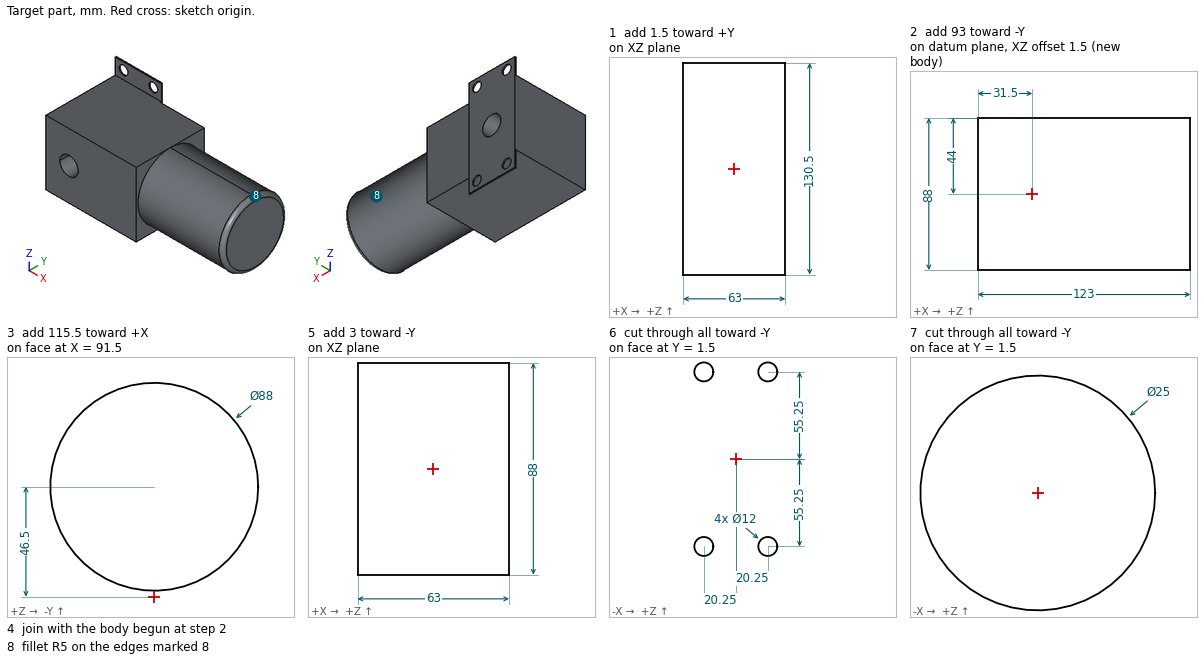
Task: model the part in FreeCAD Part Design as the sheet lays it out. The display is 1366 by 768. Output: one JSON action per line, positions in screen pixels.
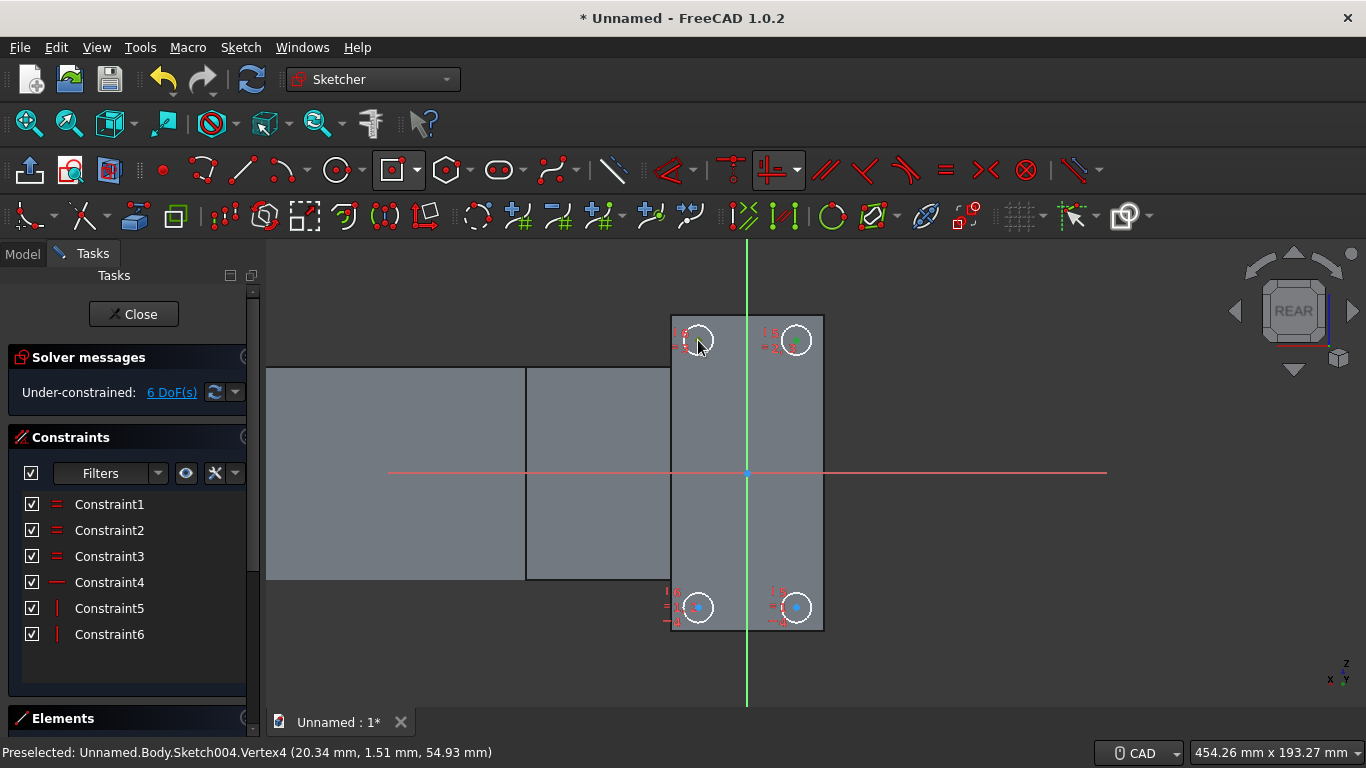
{"action": "key", "text": "h"}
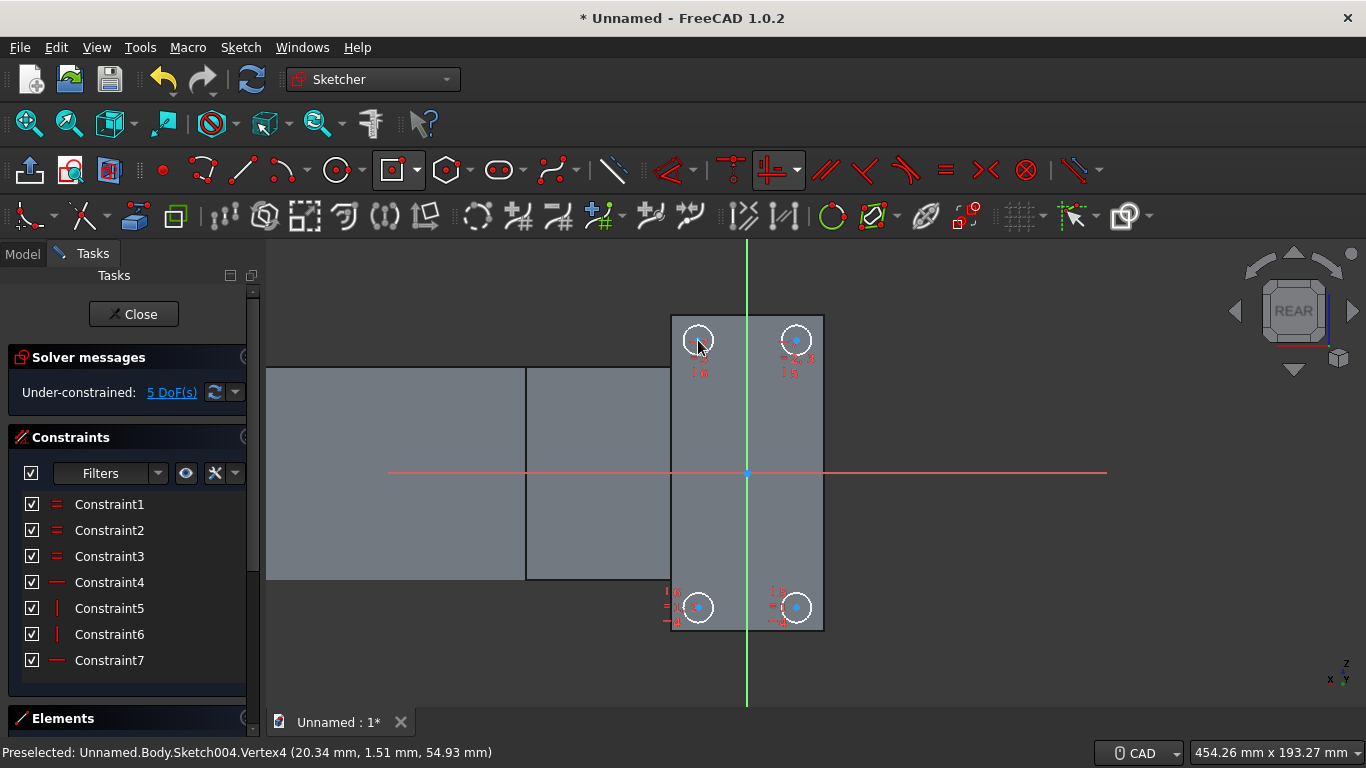
{"action": "left_click", "coordinate": [668, 170]}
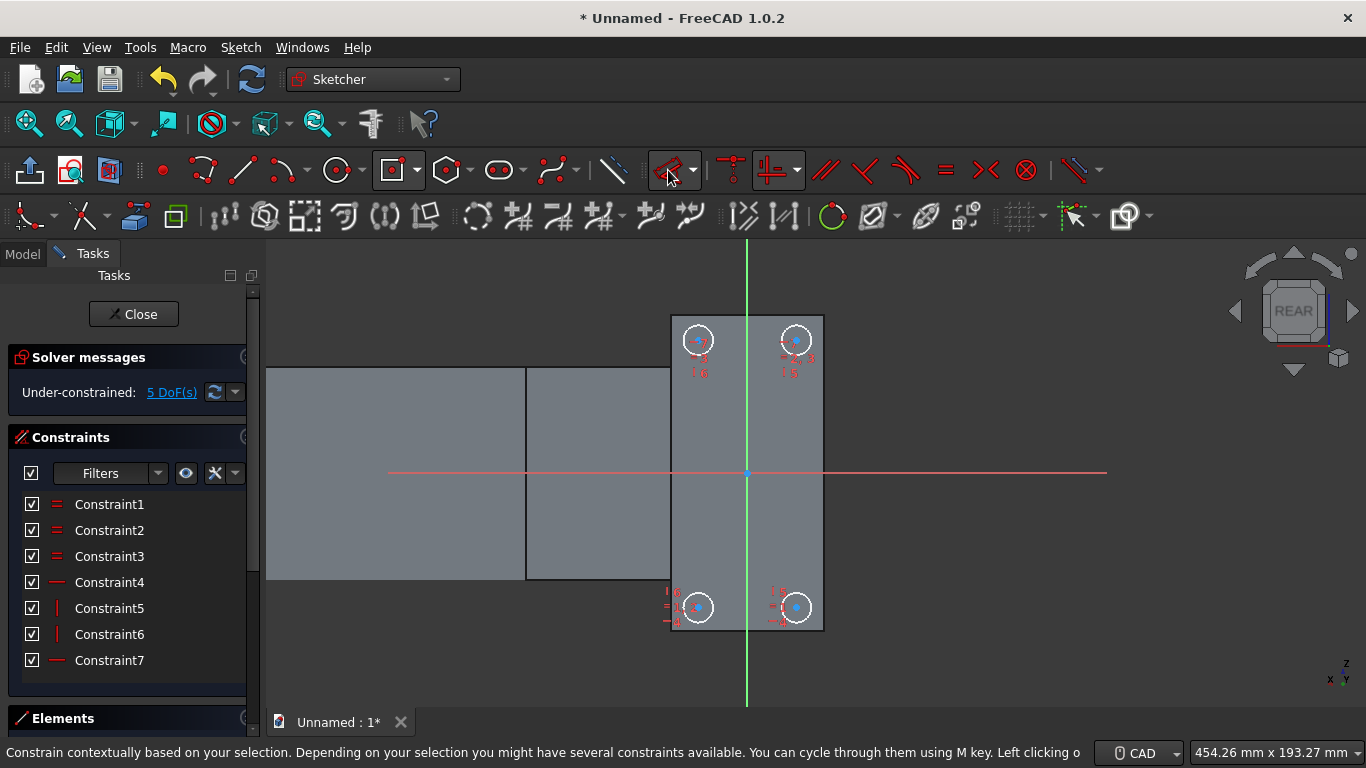
{"action": "scroll", "coordinate": [807, 597], "scroll_direction": "up", "scroll_amount": 2}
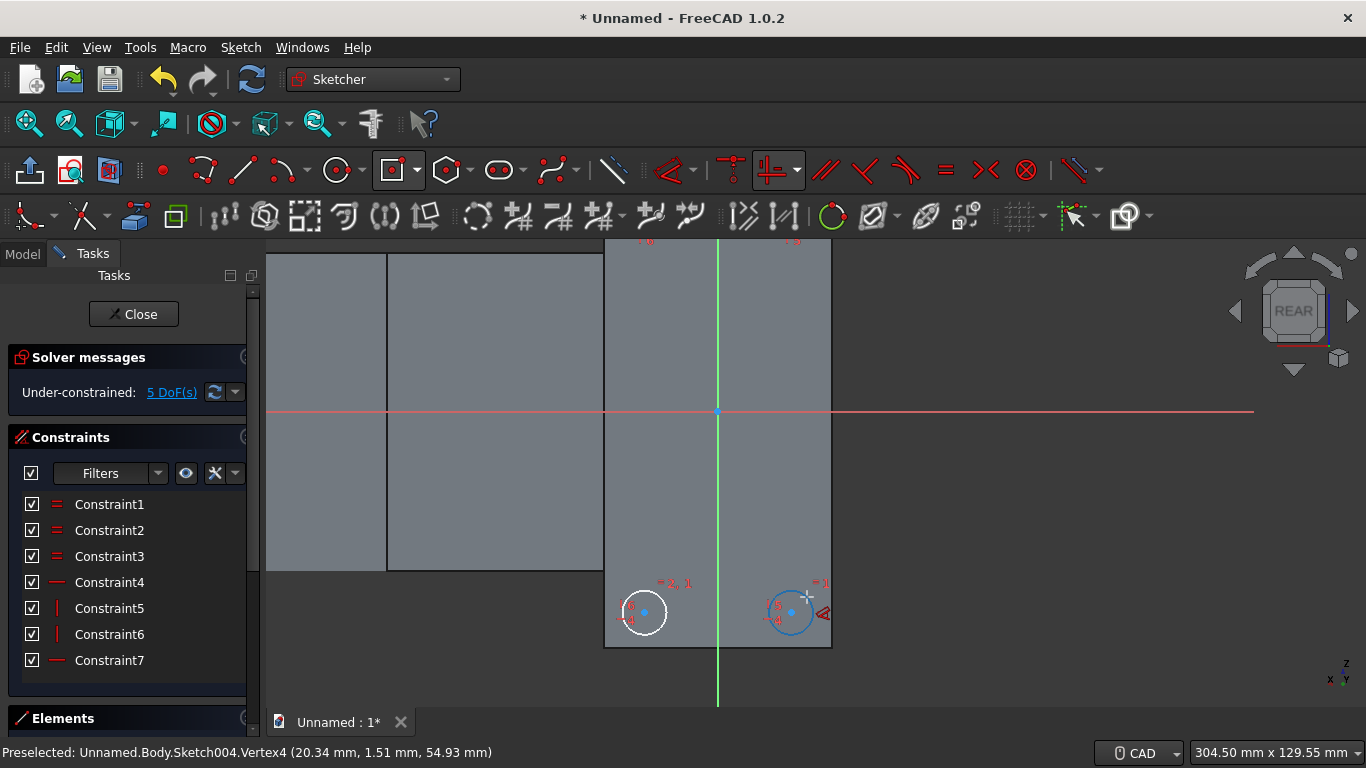
{"action": "left_click", "coordinate": [807, 597]}
{"action": "left_click", "coordinate": [830, 575]}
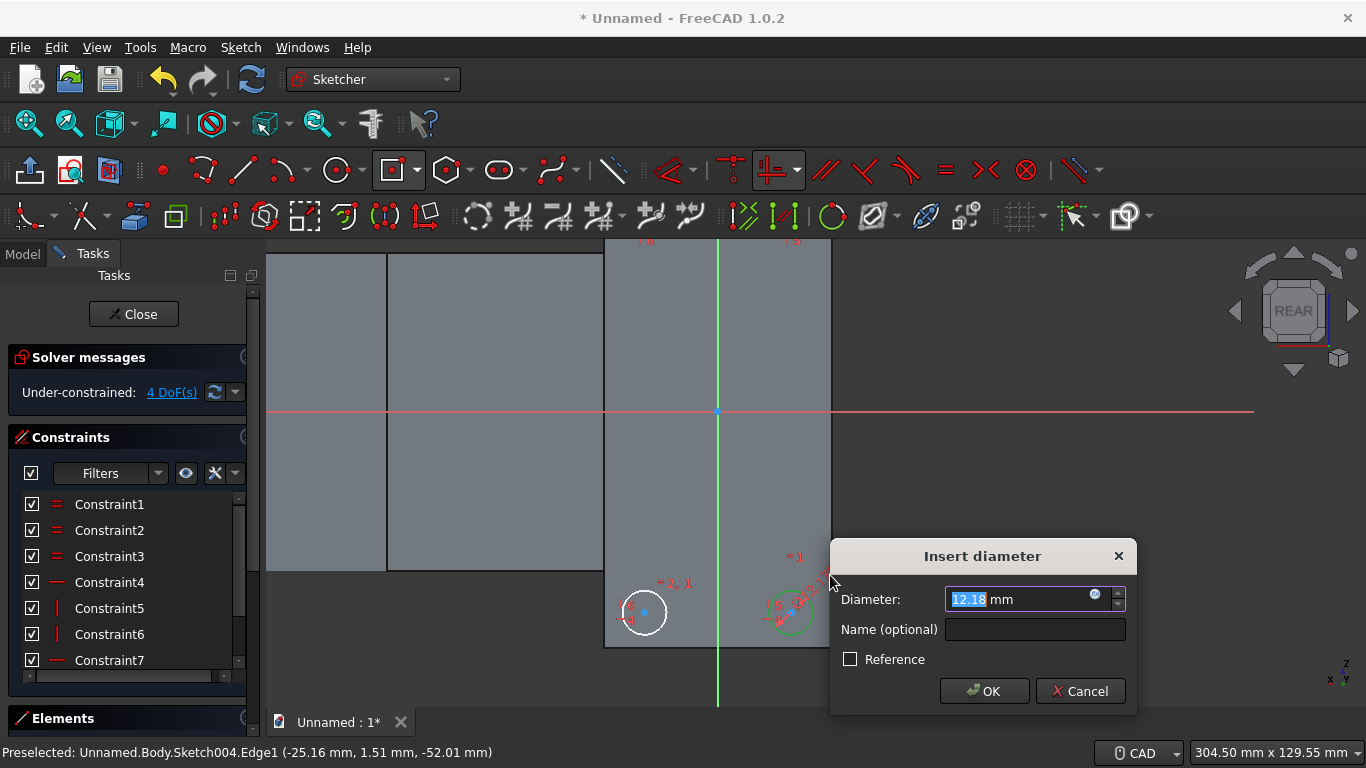
{"action": "type", "text": "12"}
{"action": "key", "text": "Return"}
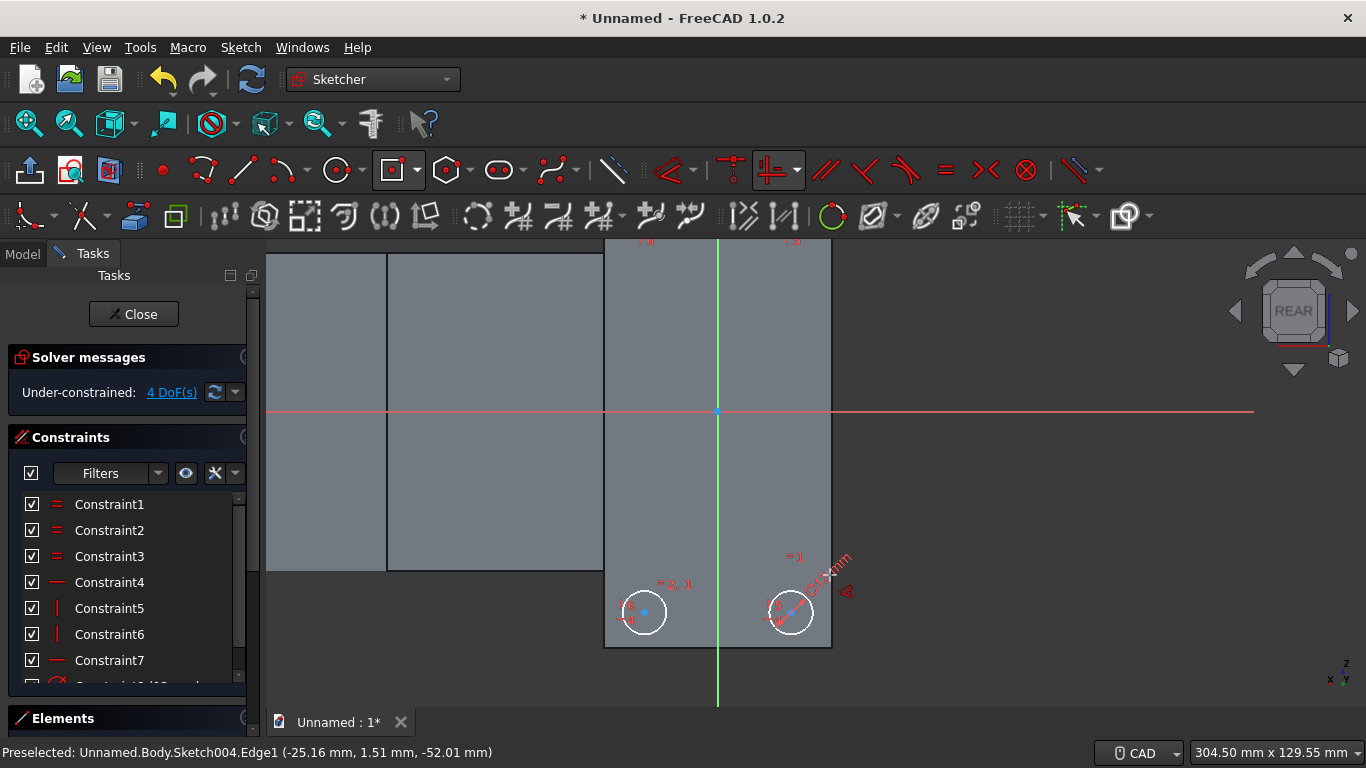
{"action": "left_click", "coordinate": [791, 613]}
{"action": "left_click", "coordinate": [755, 647]}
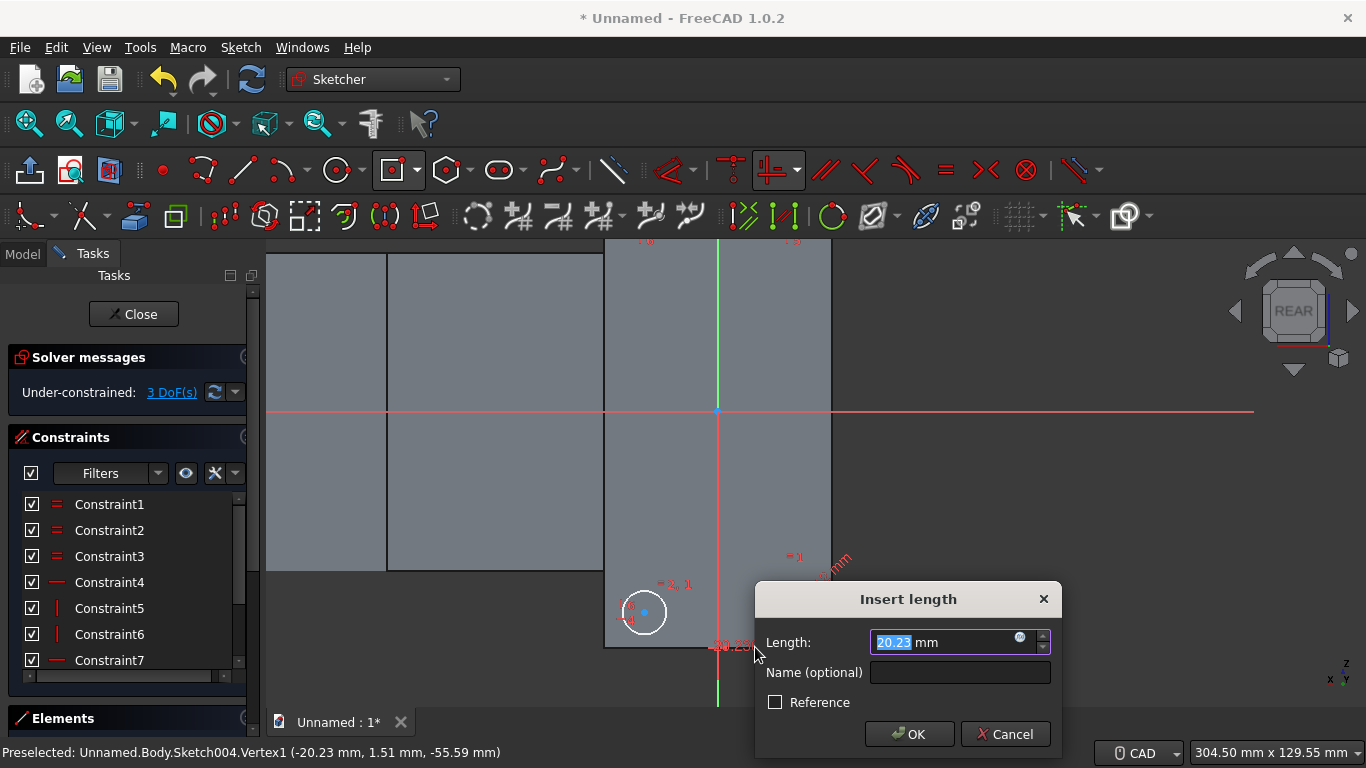
{"action": "type", "text": "20.25"}
{"action": "key", "text": "Return"}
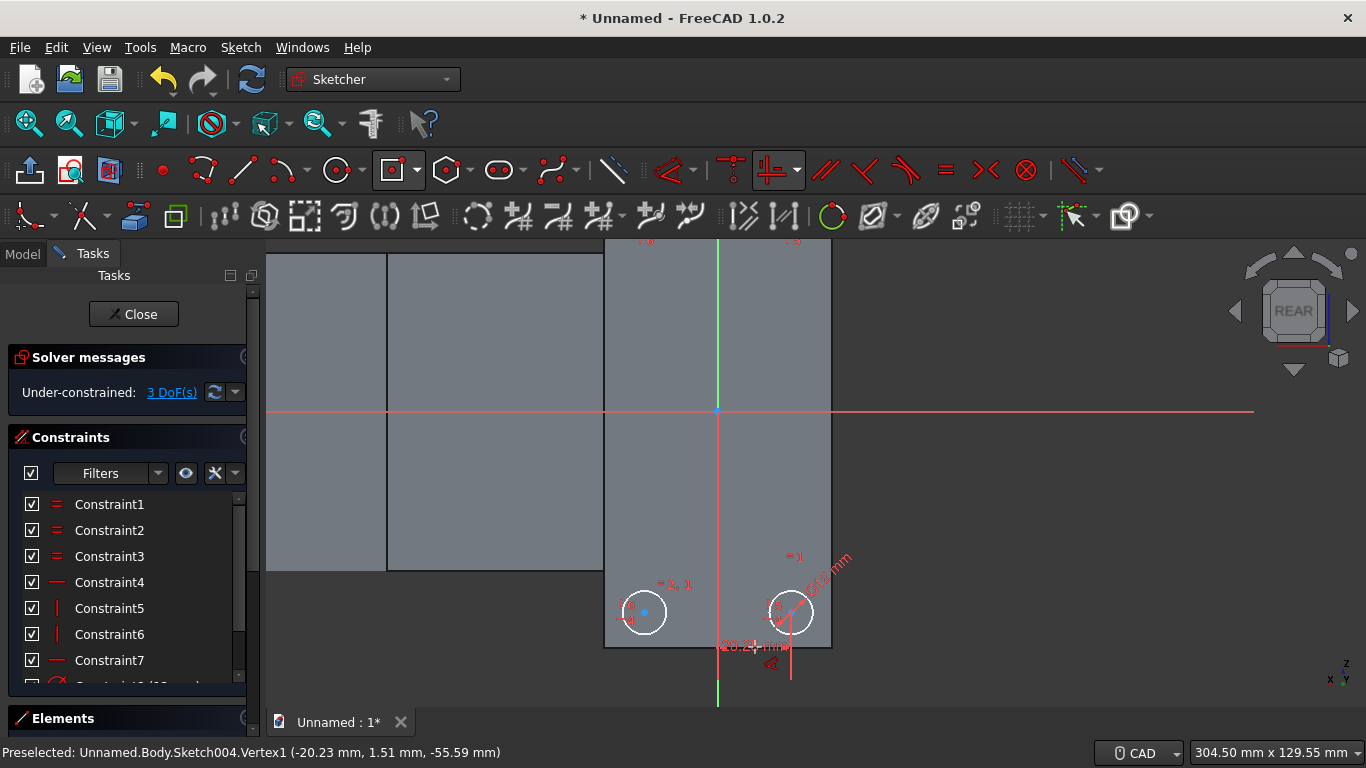
{"action": "left_click", "coordinate": [791, 613]}
{"action": "left_click", "coordinate": [825, 512]}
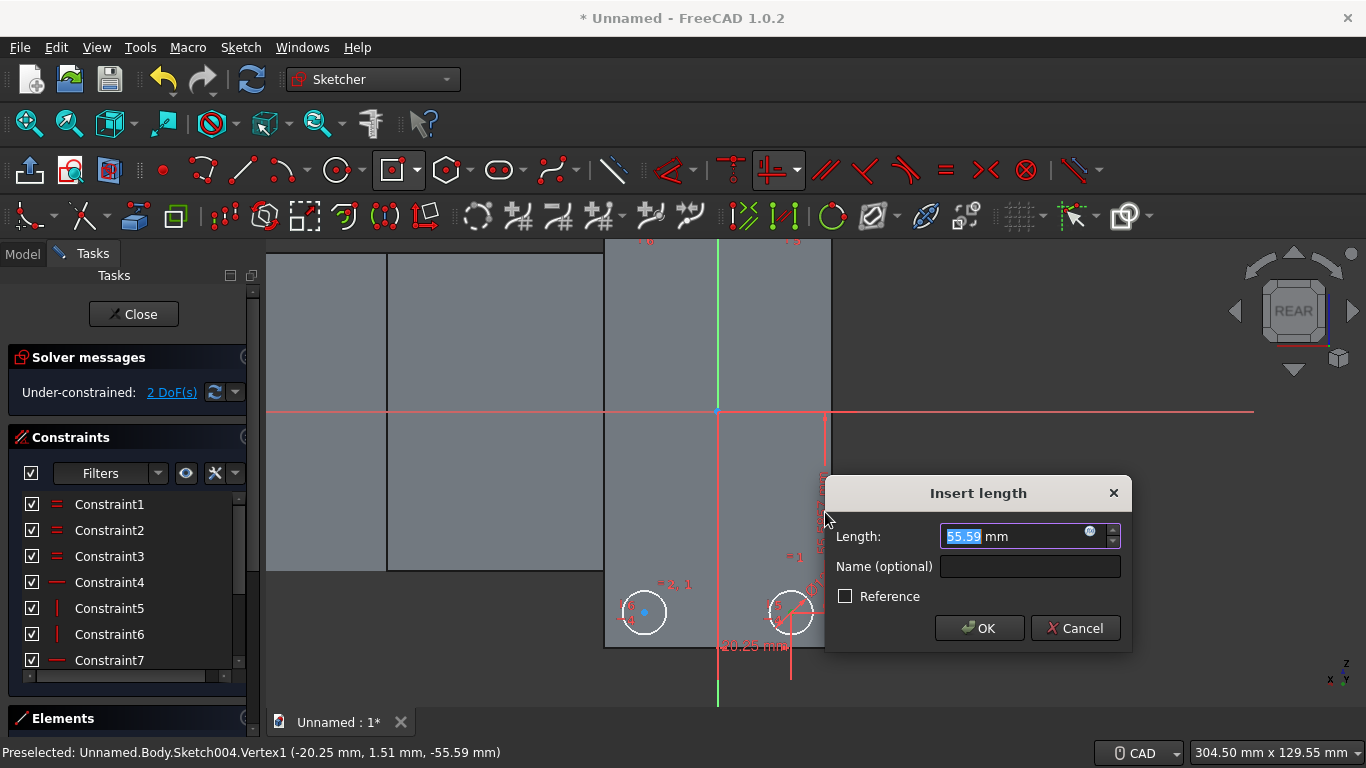
{"action": "type", "text": "55.25"}
{"action": "key", "text": "Return"}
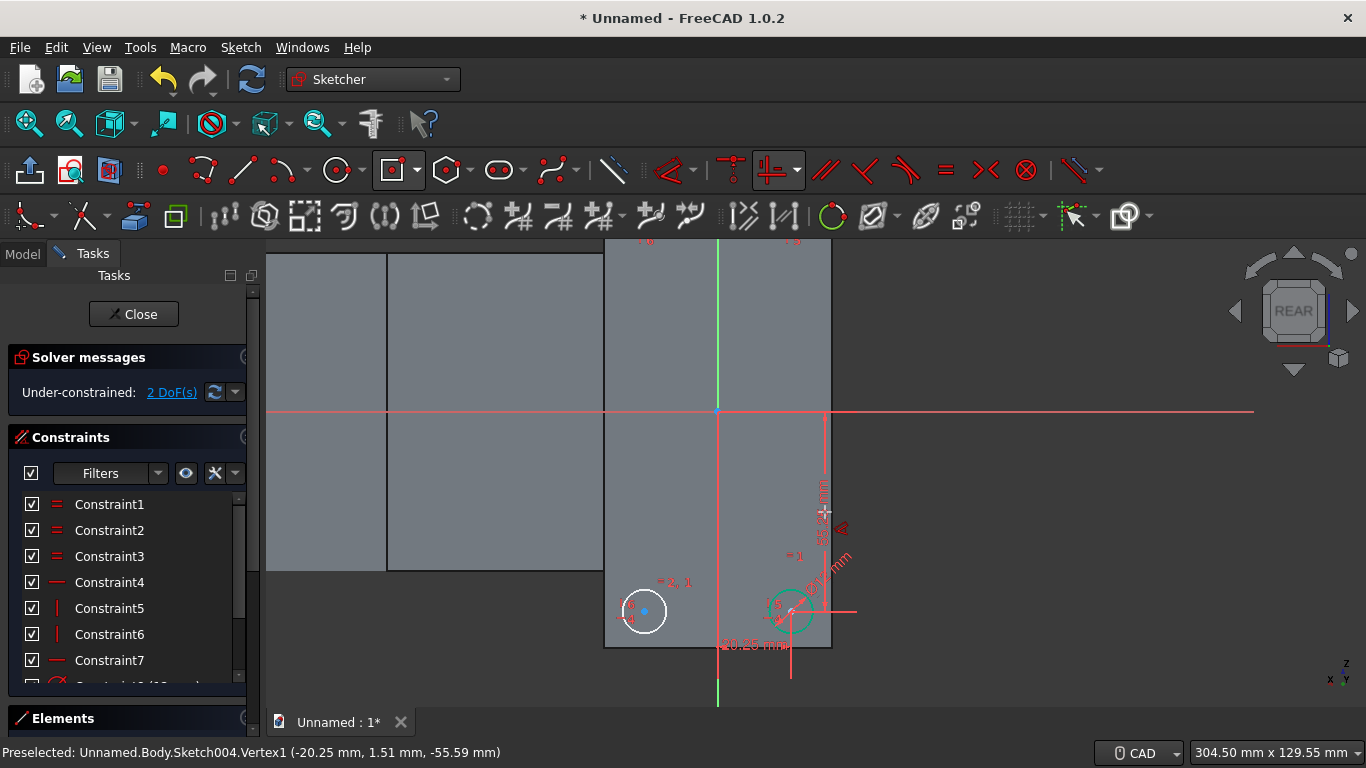
{"action": "left_click", "coordinate": [645, 612]}
{"action": "left_click", "coordinate": [681, 646]}